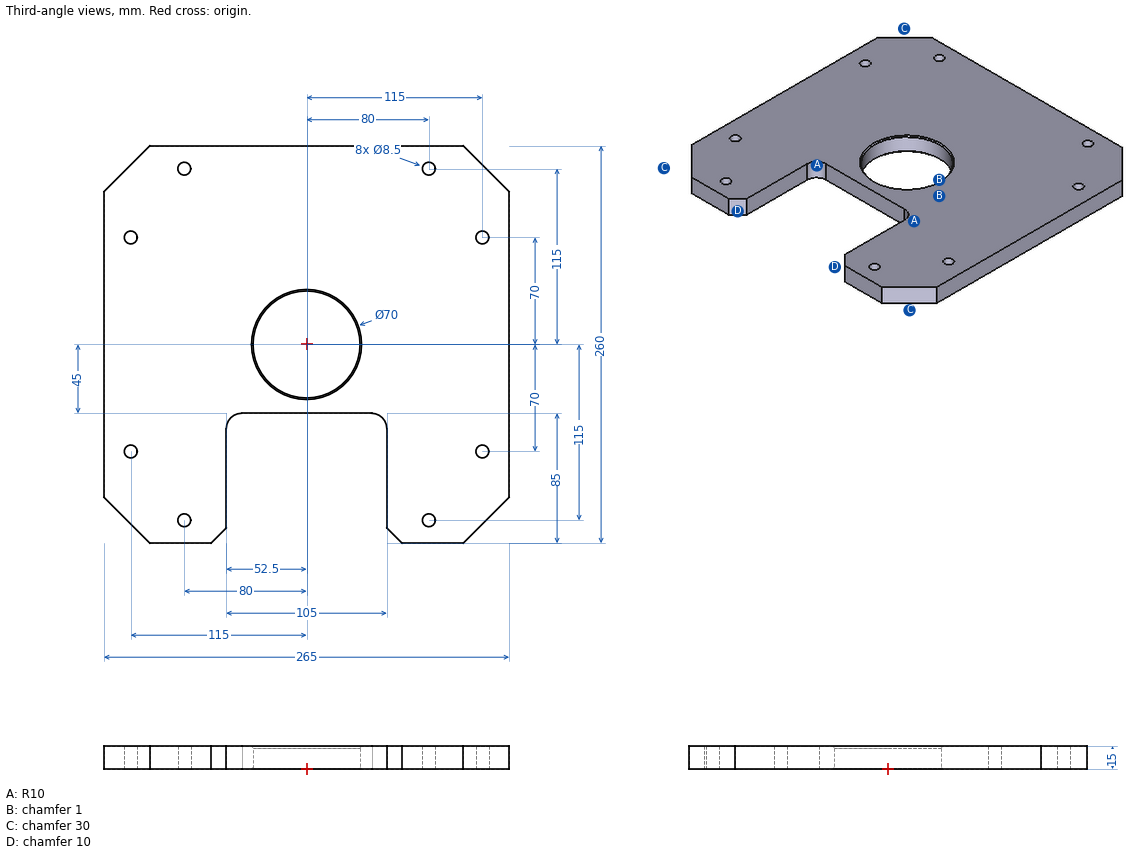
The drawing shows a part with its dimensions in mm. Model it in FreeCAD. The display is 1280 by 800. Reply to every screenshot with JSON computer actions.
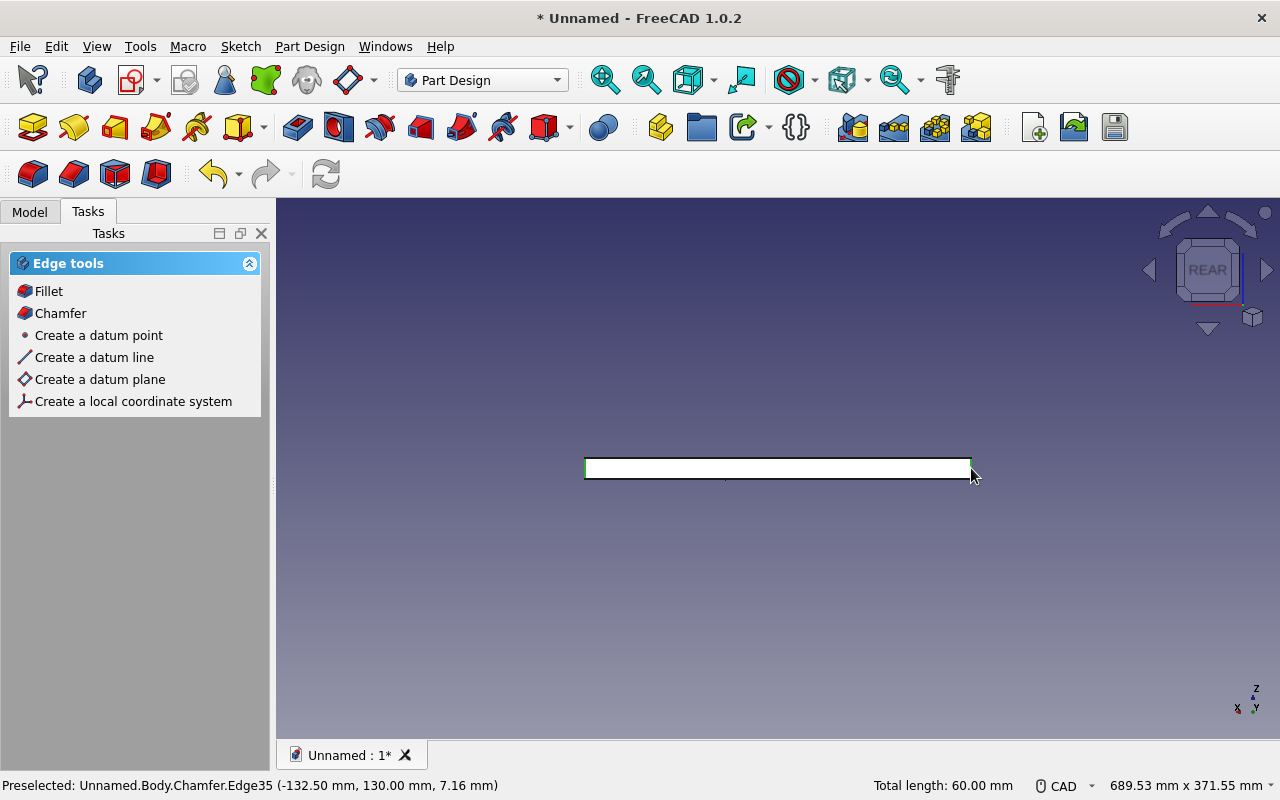
{"action": "left_click", "coordinate": [74, 174]}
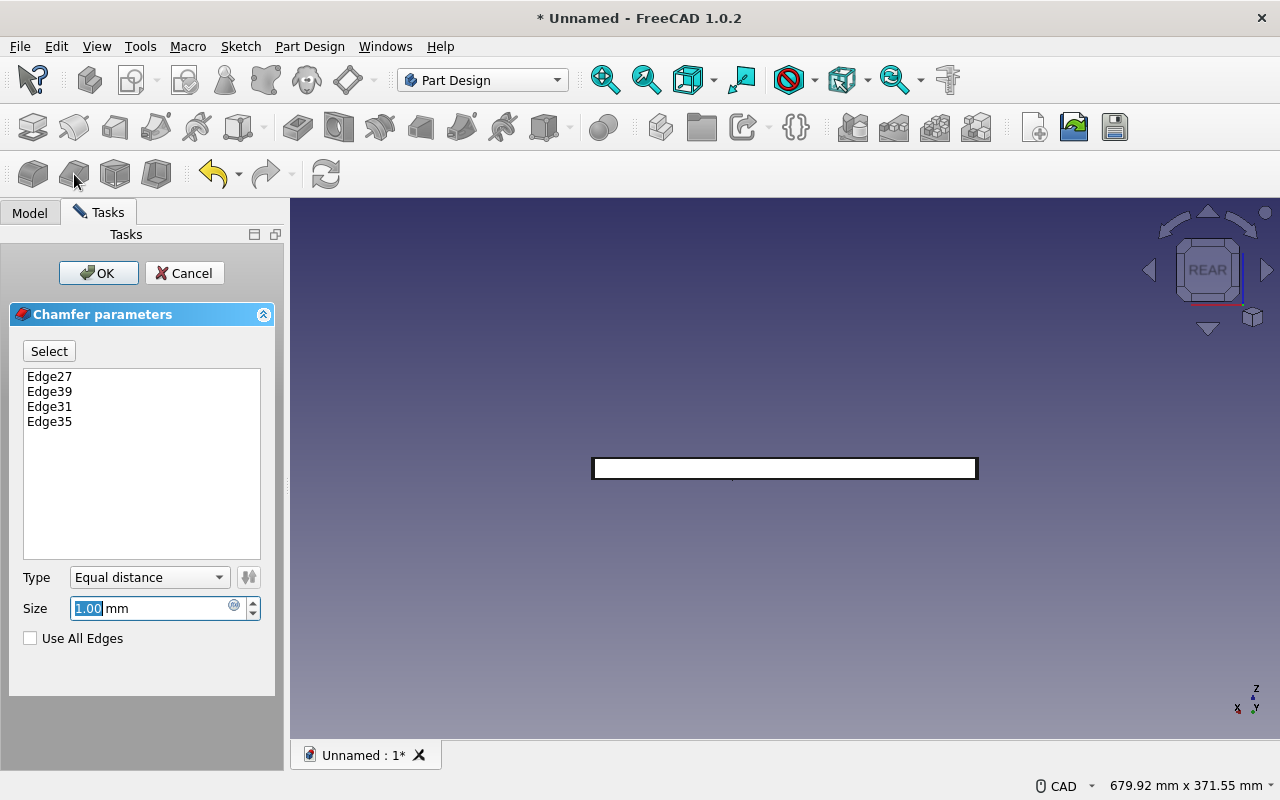
{"action": "type", "text": "30"}
{"action": "key", "text": "Tab"}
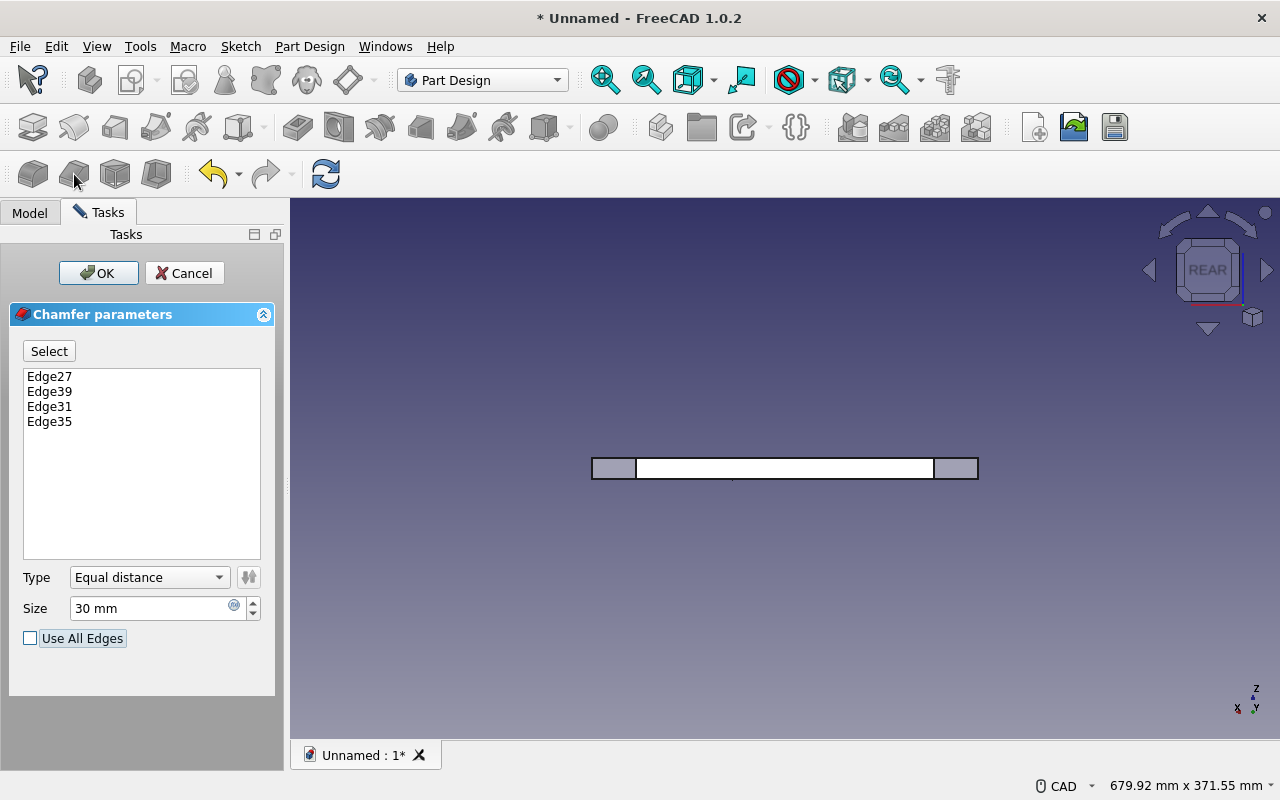
{"action": "left_click", "coordinate": [99, 273]}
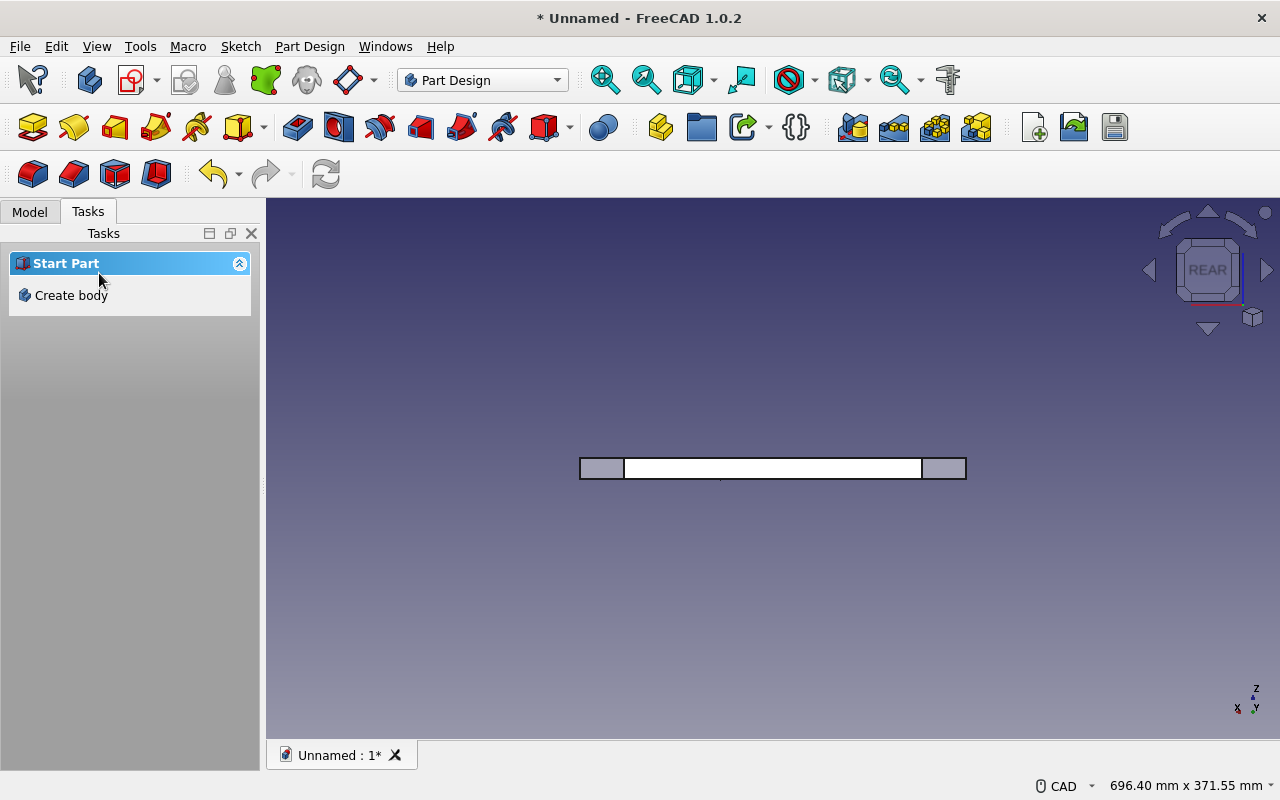
{"action": "left_click", "coordinate": [606, 80]}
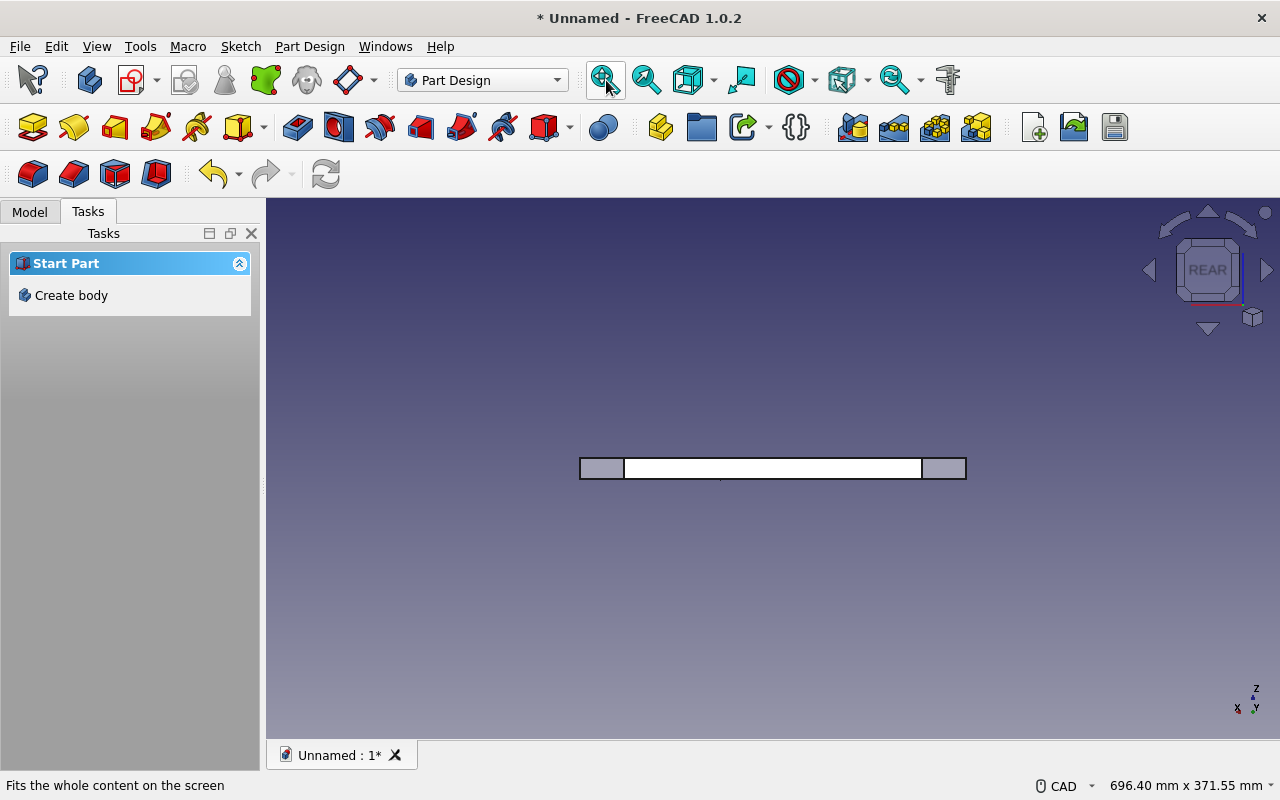
{"action": "scroll", "coordinate": [697, 468], "scroll_direction": "up", "scroll_amount": 4}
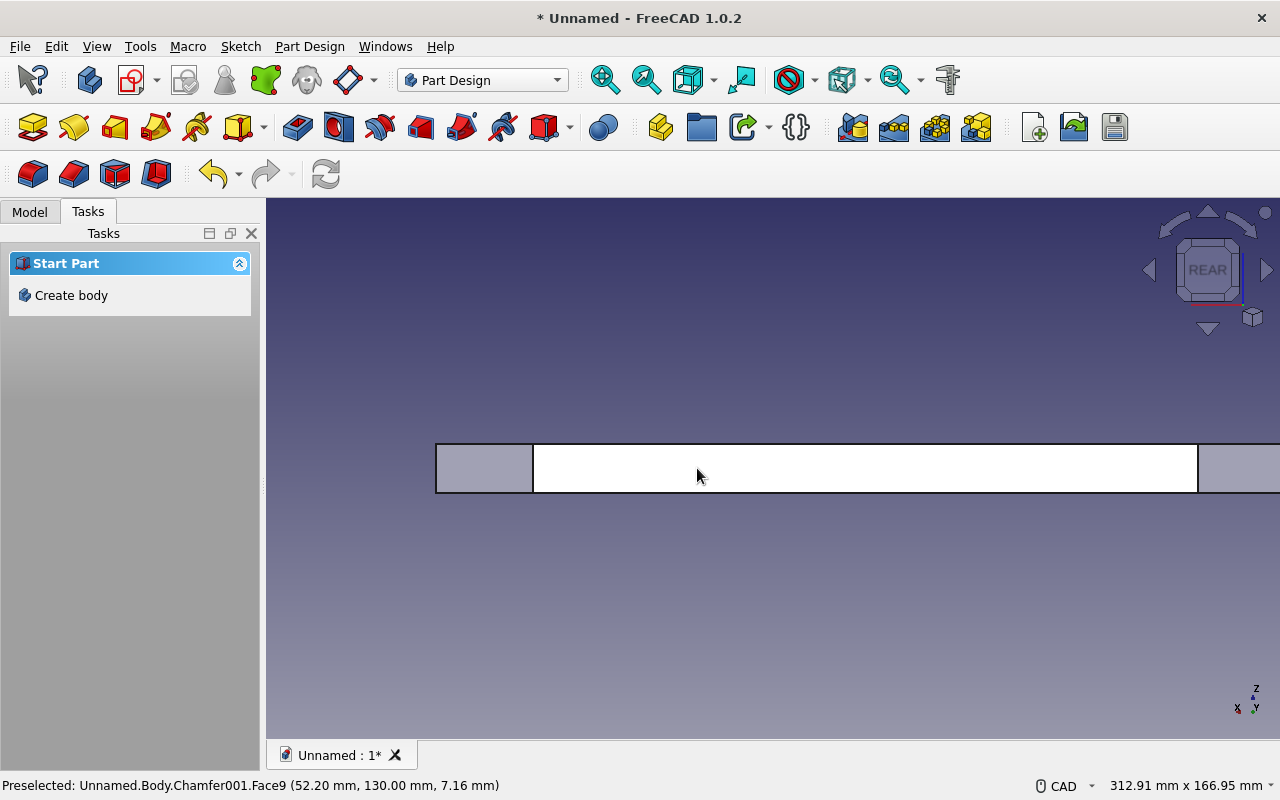
{"action": "key", "text": "v f"}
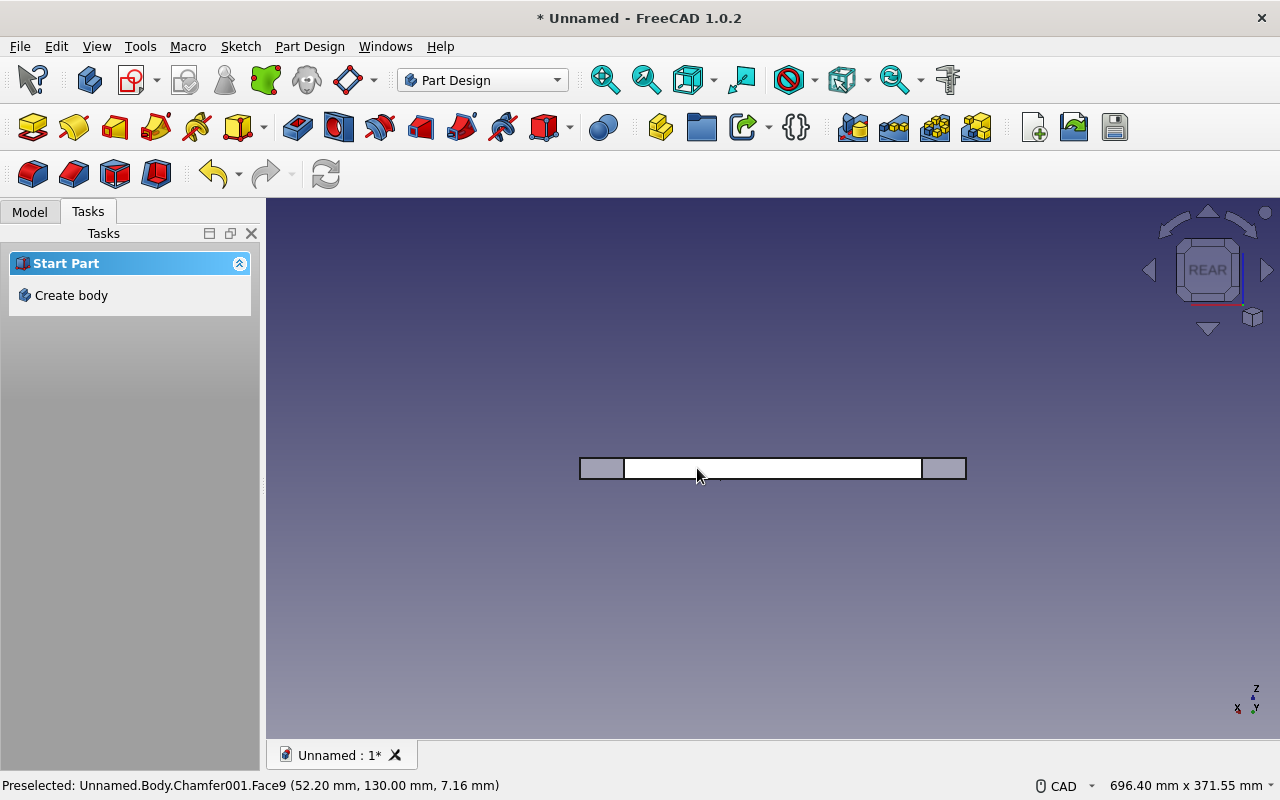
{"action": "key", "text": "0"}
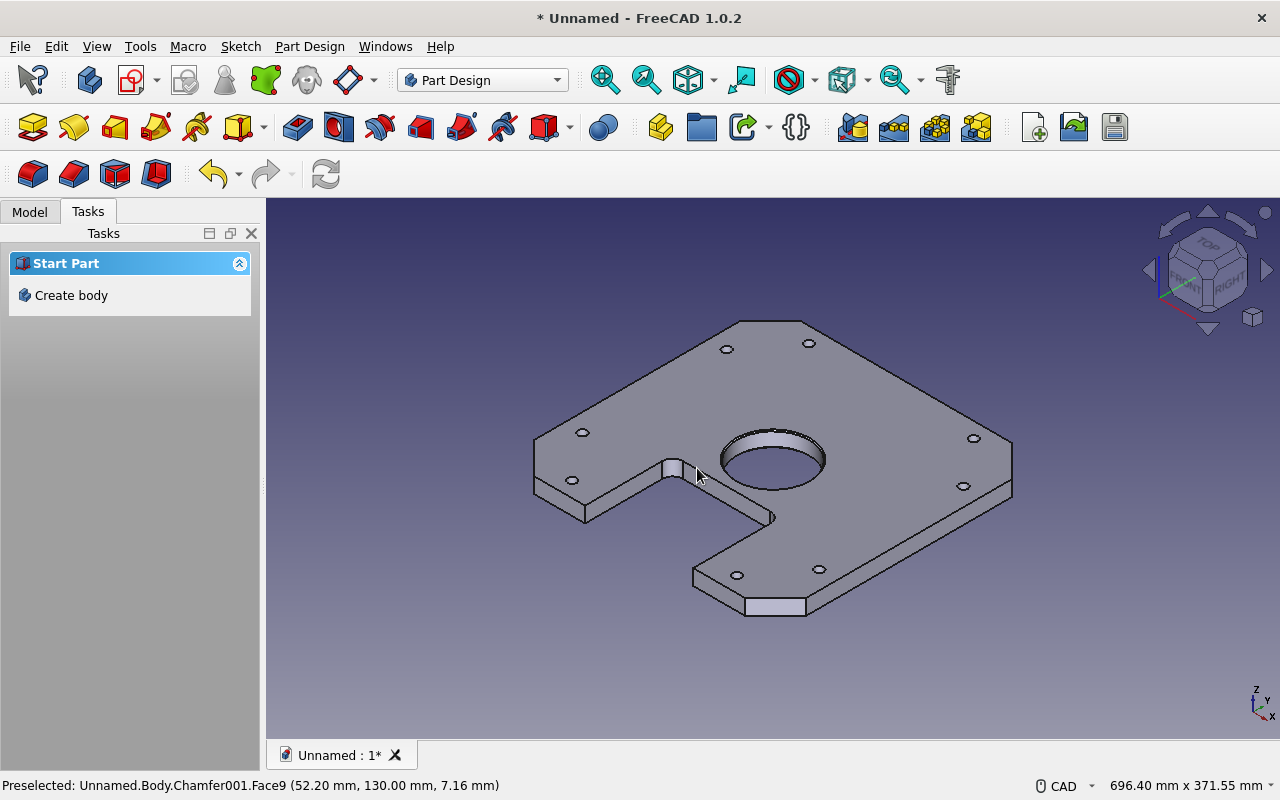
{"action": "left_click", "coordinate": [585, 514]}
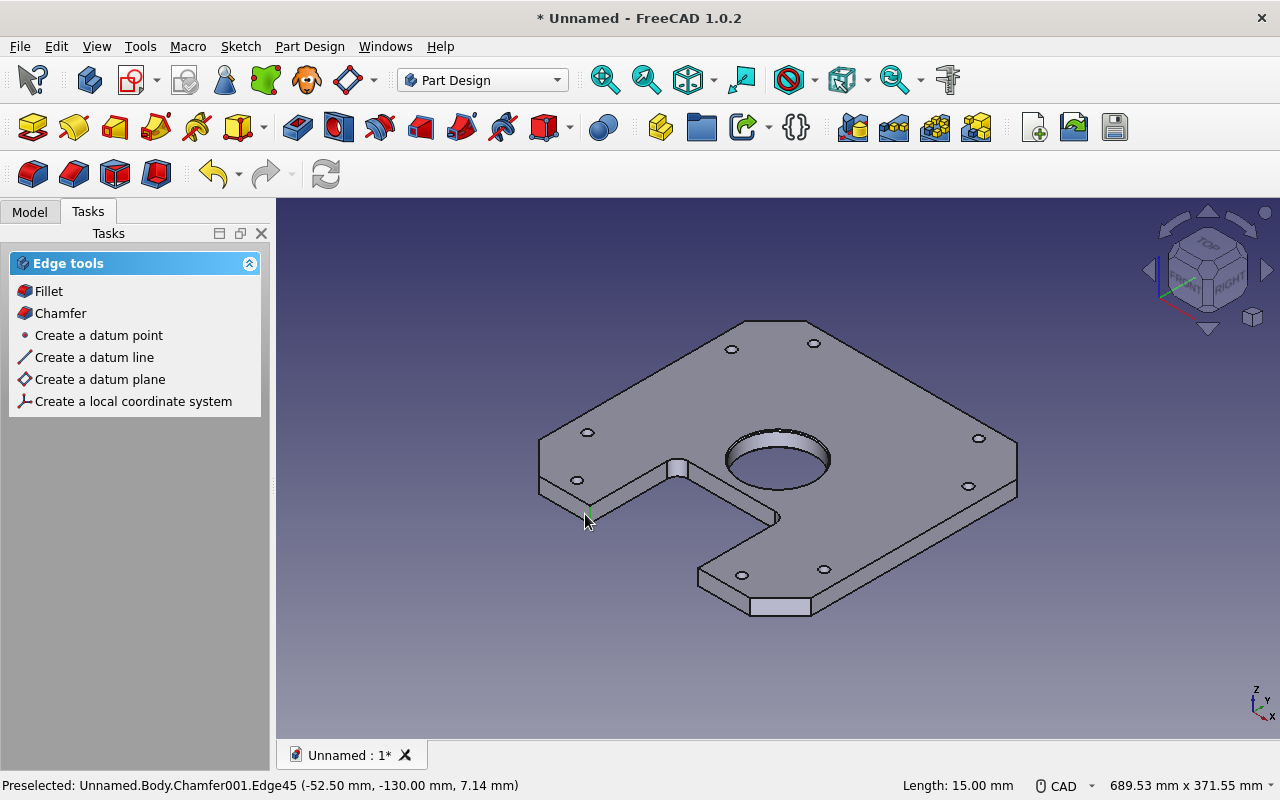
{"action": "scroll", "coordinate": [698, 576], "scroll_direction": "up", "scroll_amount": 4}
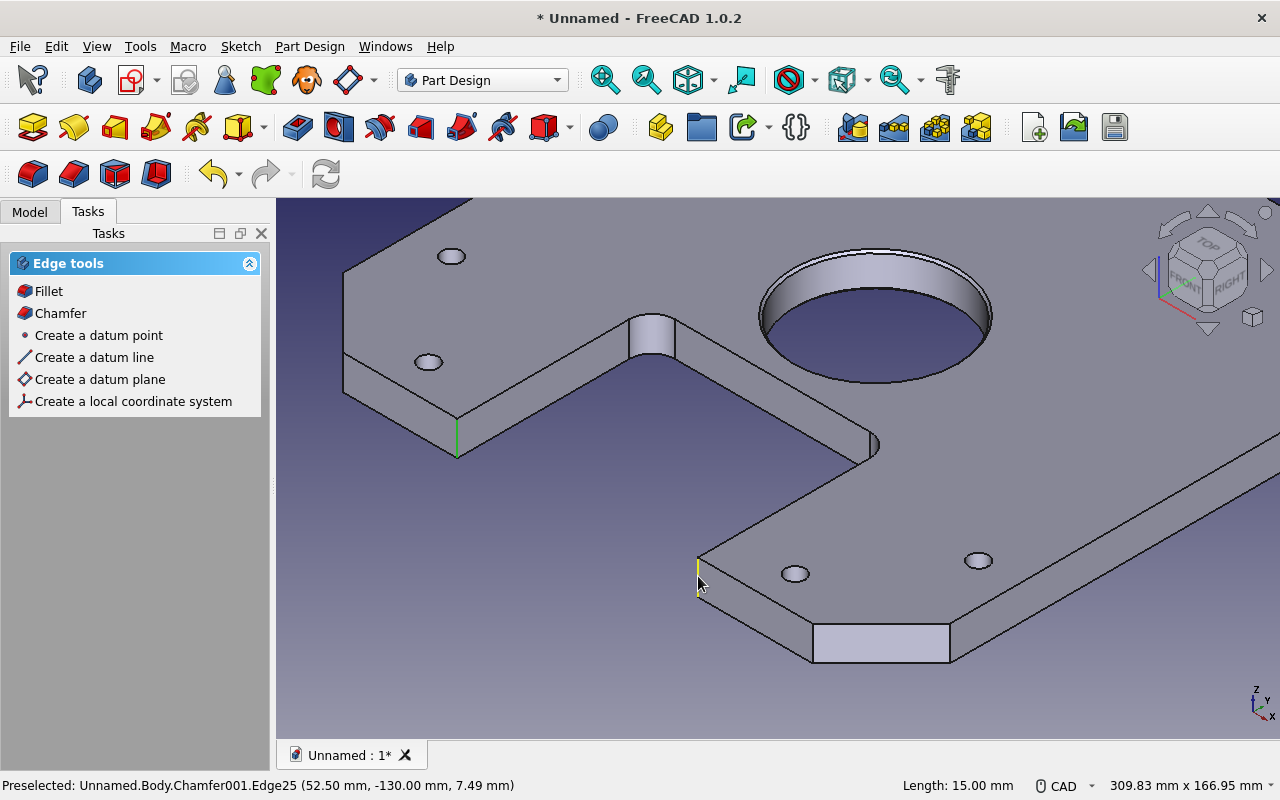
{"action": "left_click", "coordinate": [606, 80]}